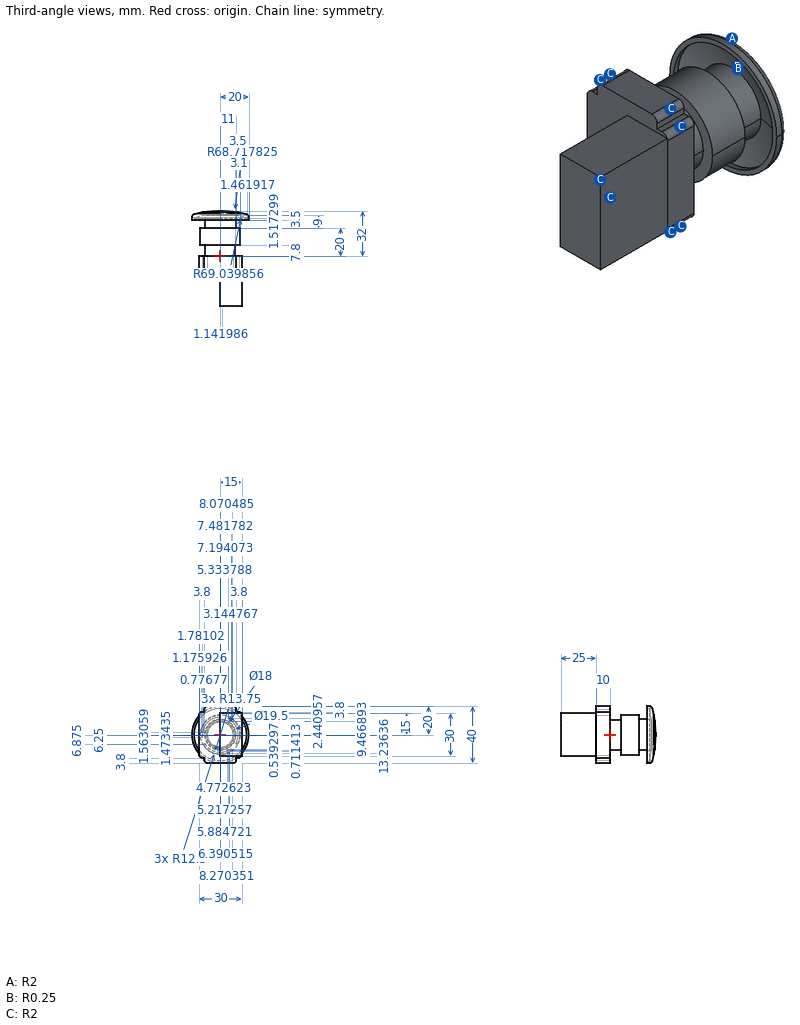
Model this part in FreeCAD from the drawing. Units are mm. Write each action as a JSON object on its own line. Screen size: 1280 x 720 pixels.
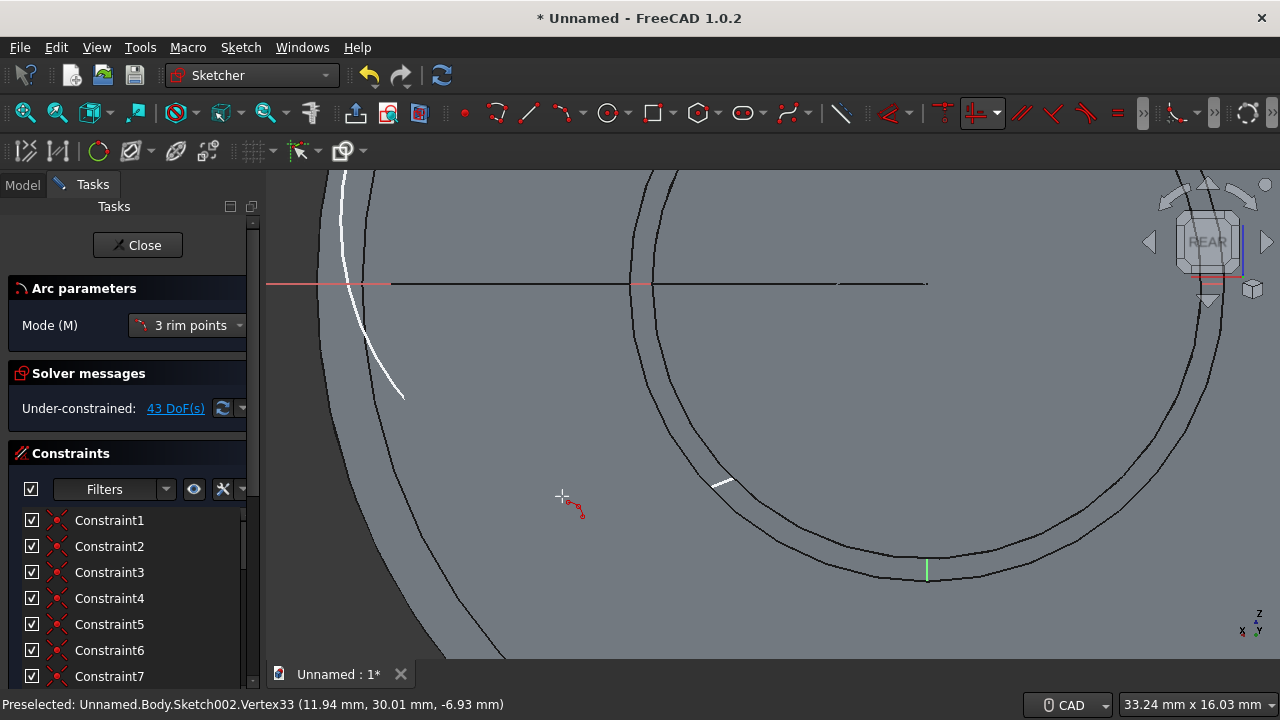
{"action": "scroll", "coordinate": [563, 495], "scroll_direction": "down", "scroll_amount": 5}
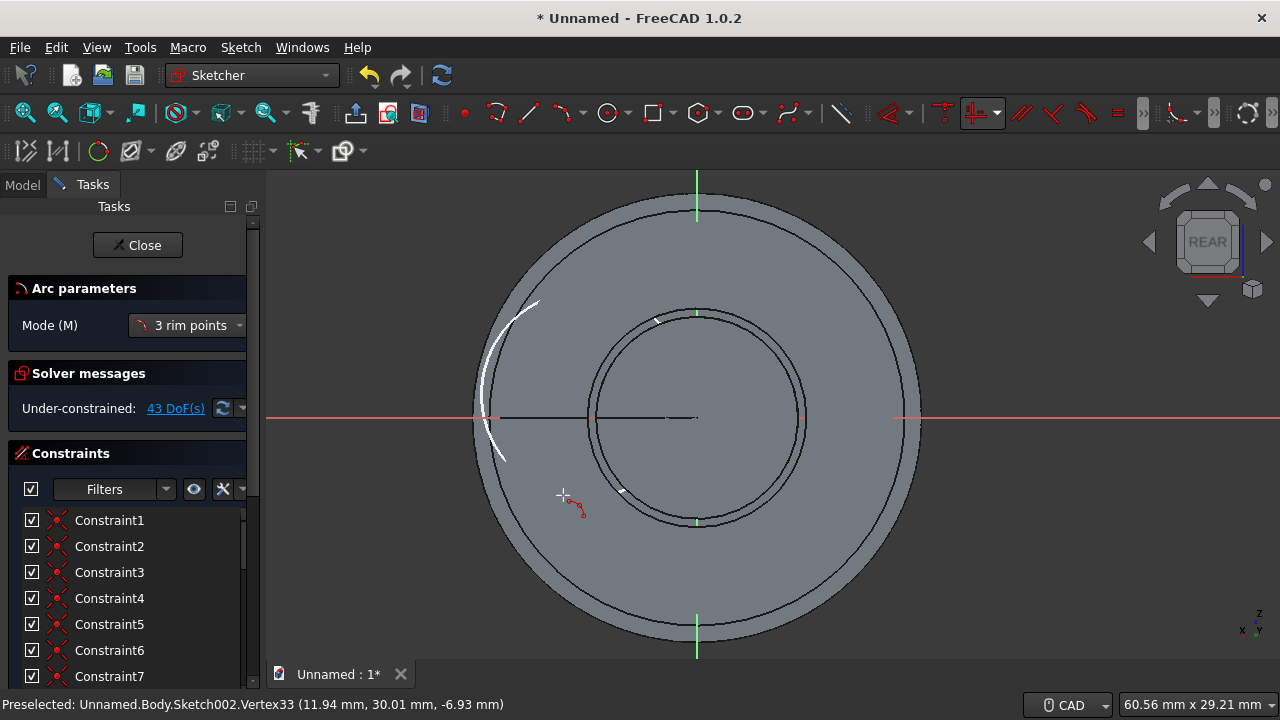
{"action": "left_click", "coordinate": [546, 386]}
{"action": "key", "text": "Escape"}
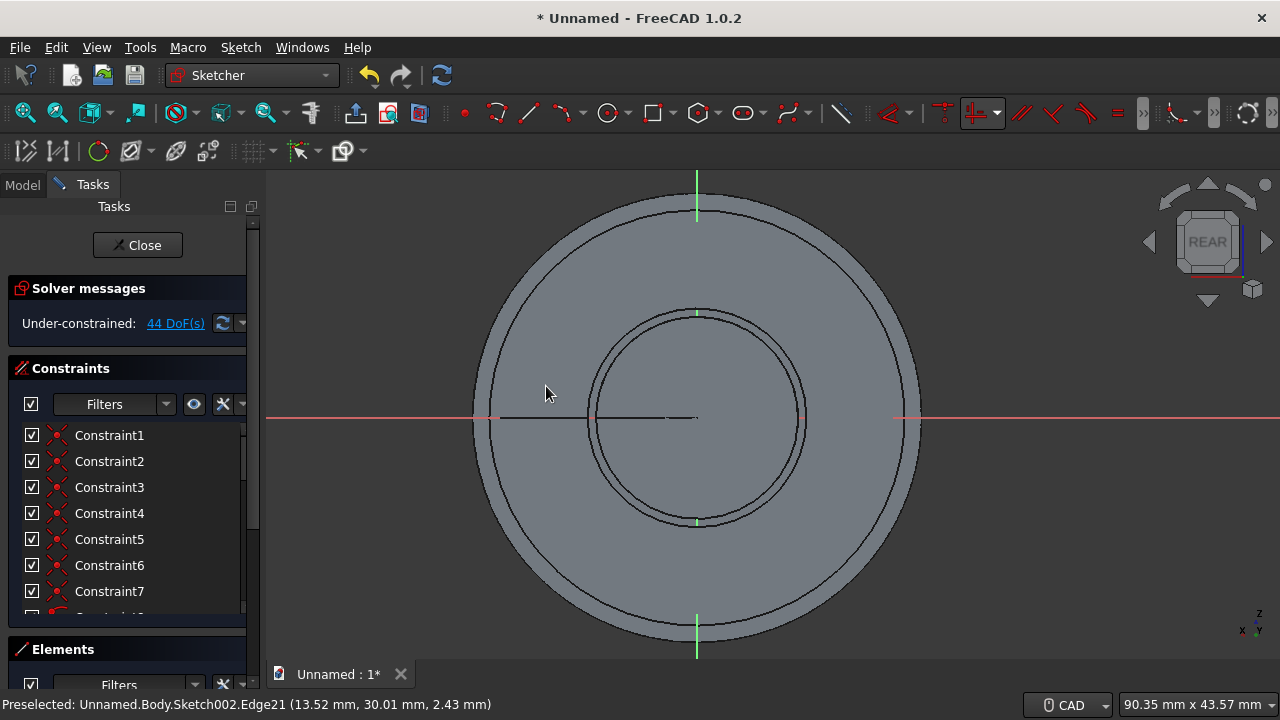
{"action": "scroll", "coordinate": [701, 270], "scroll_direction": "up", "scroll_amount": 5}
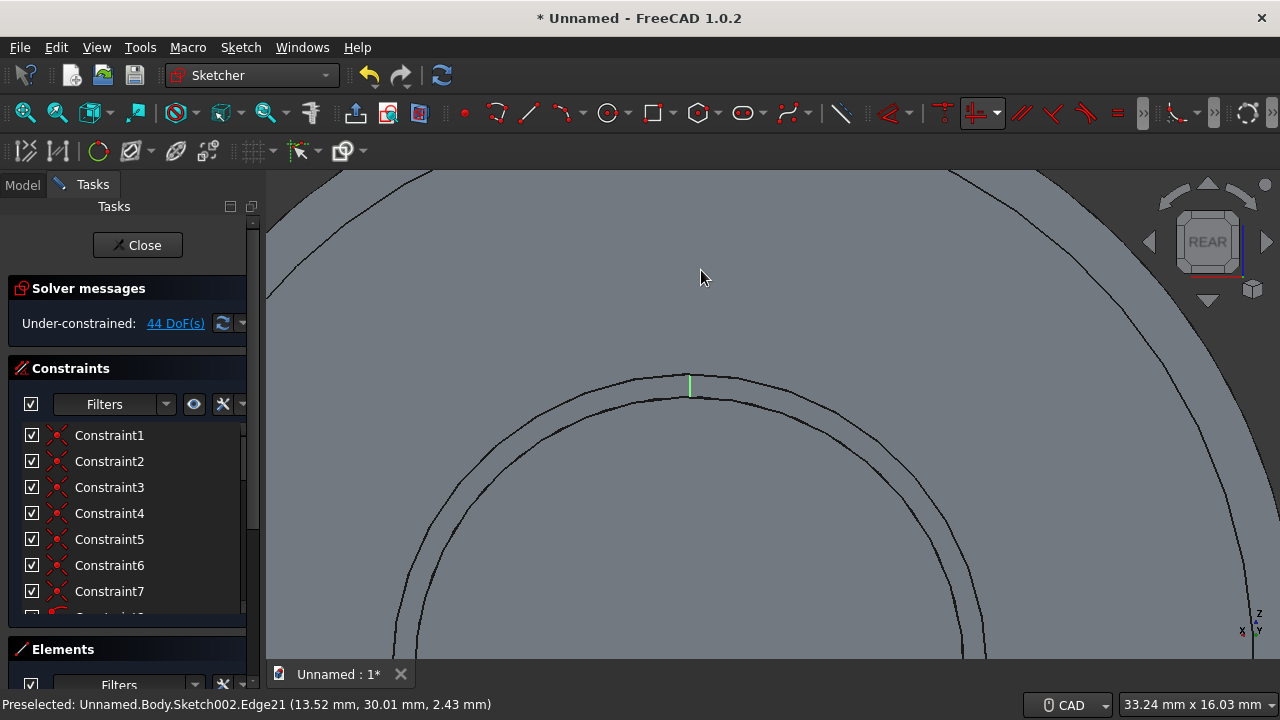
{"action": "left_click", "coordinate": [699, 269]}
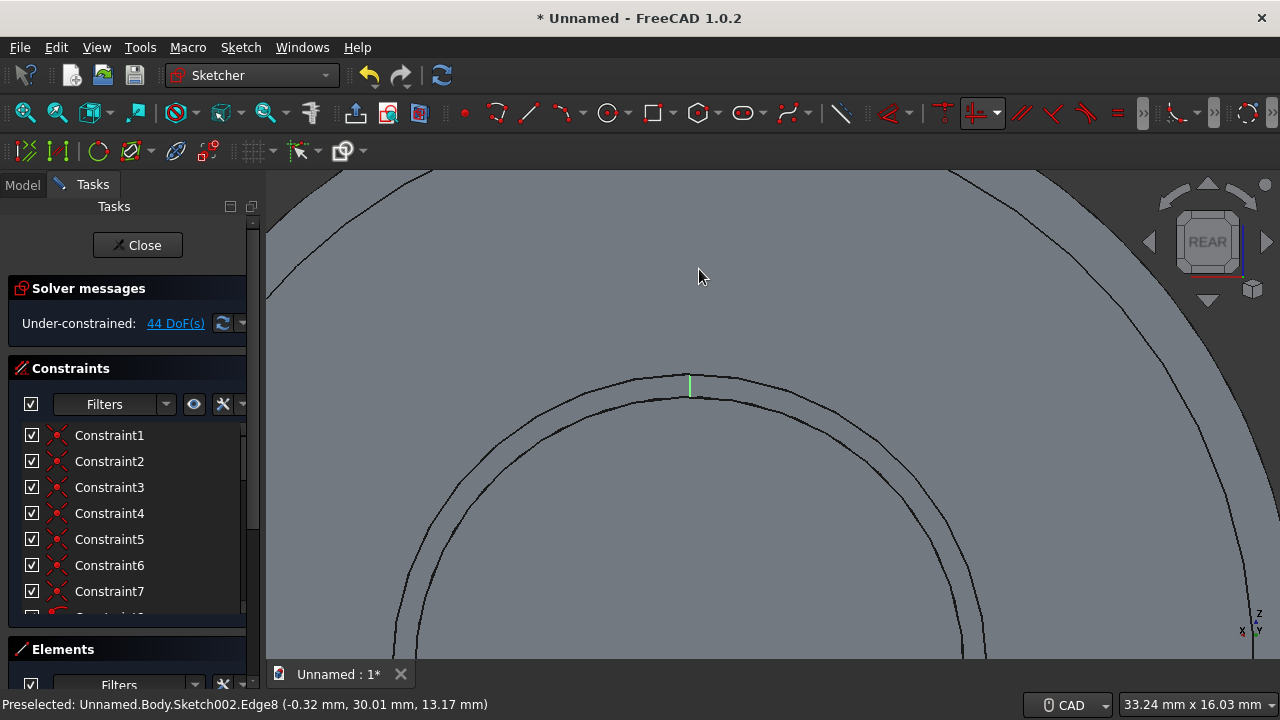
{"action": "left_click", "coordinate": [1000, 114]}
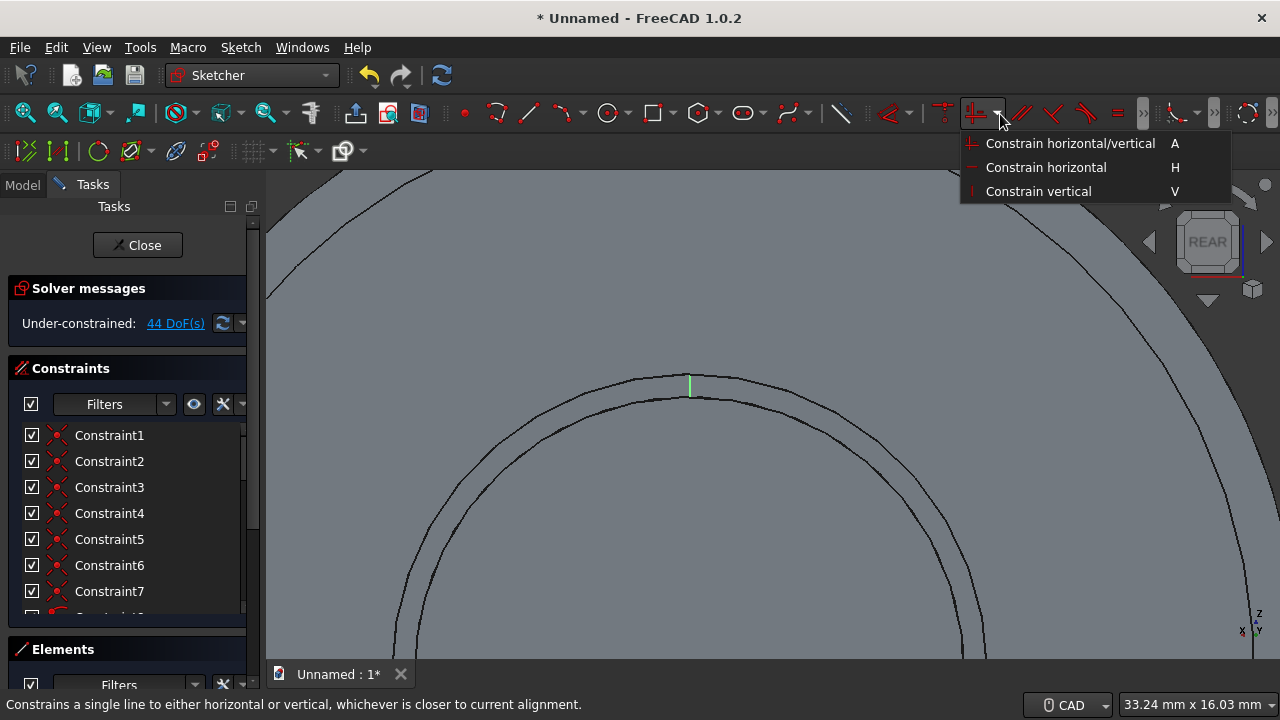
{"action": "left_click", "coordinate": [1096, 191]}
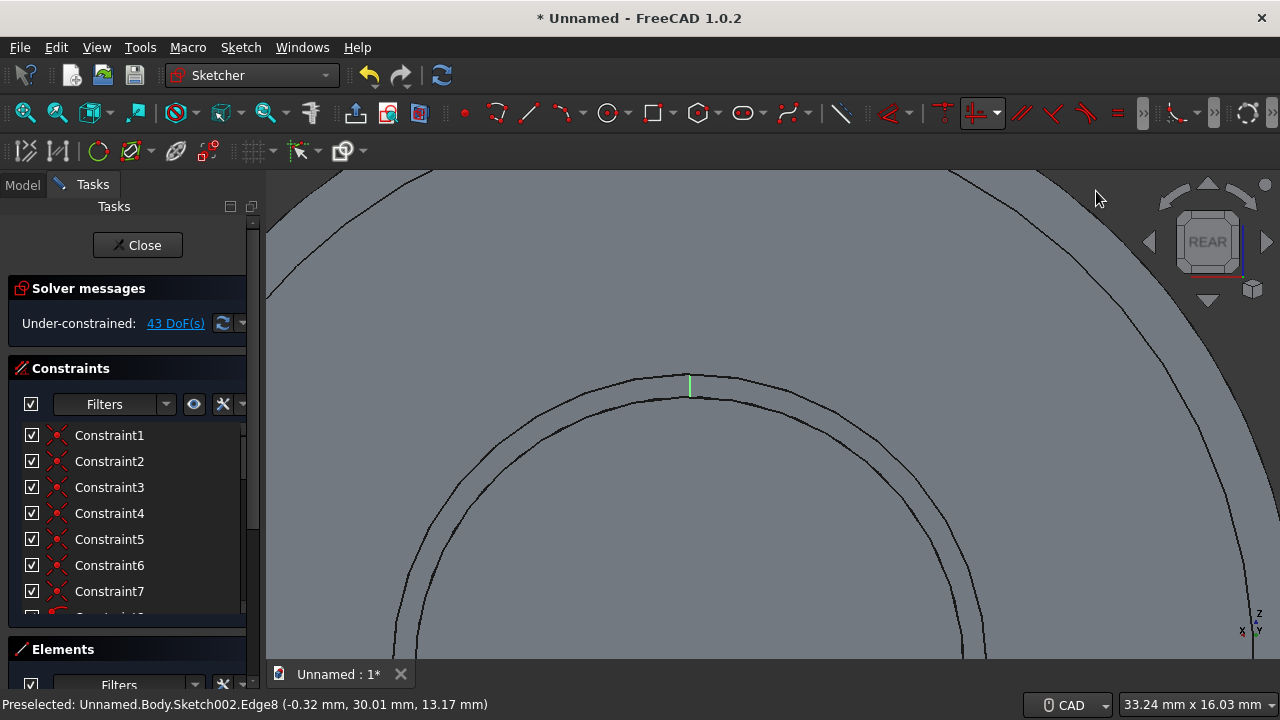
{"action": "scroll", "coordinate": [701, 269], "scroll_direction": "down", "scroll_amount": 5}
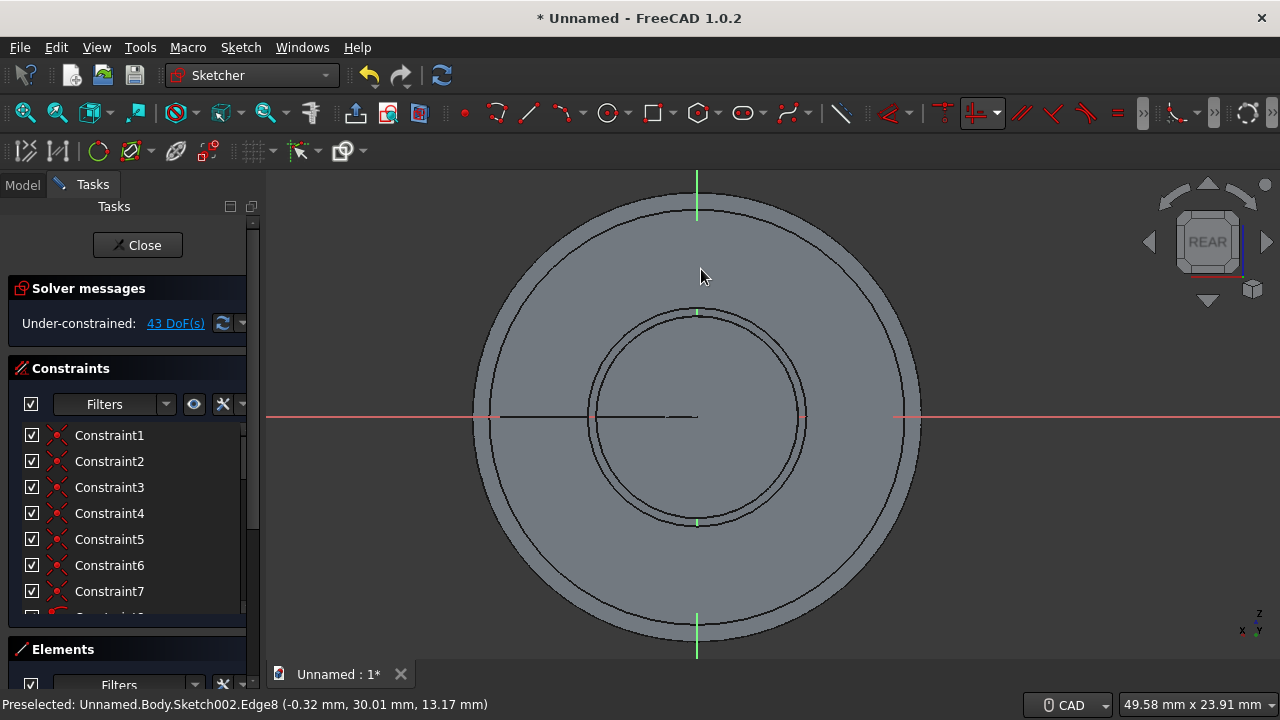
{"action": "left_click", "coordinate": [776, 534]}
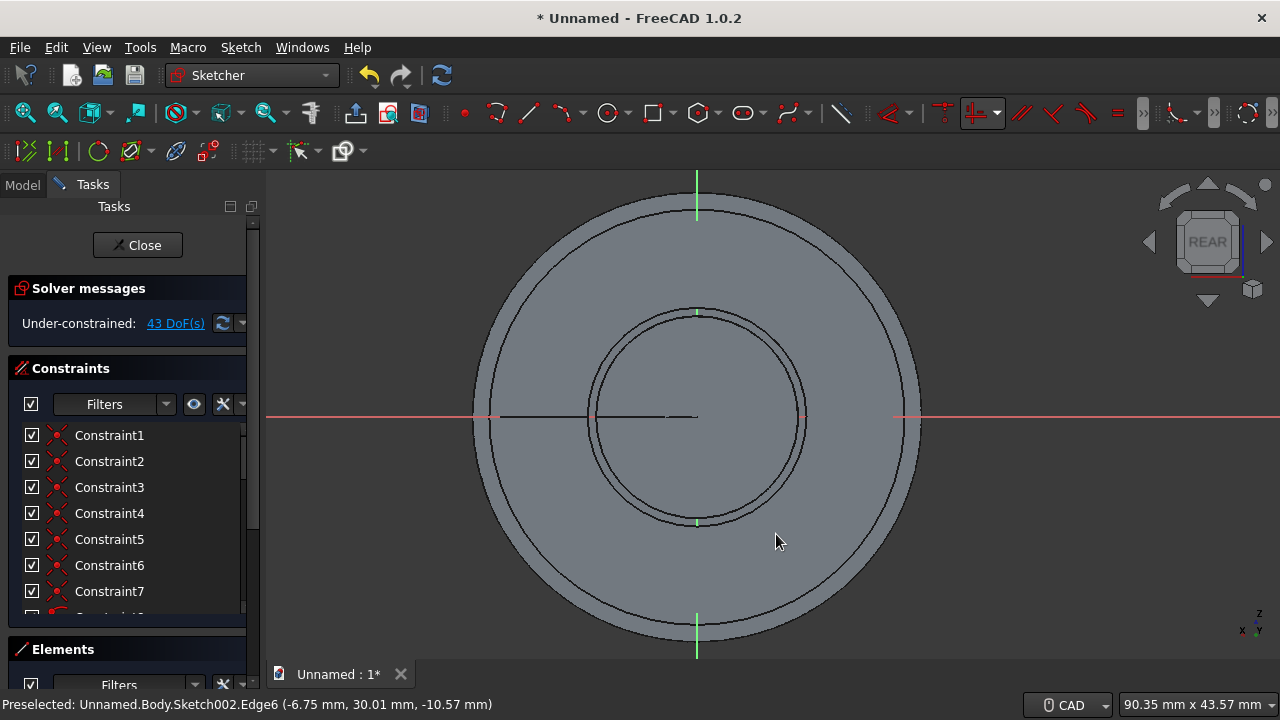
{"action": "left_click", "coordinate": [697, 572]}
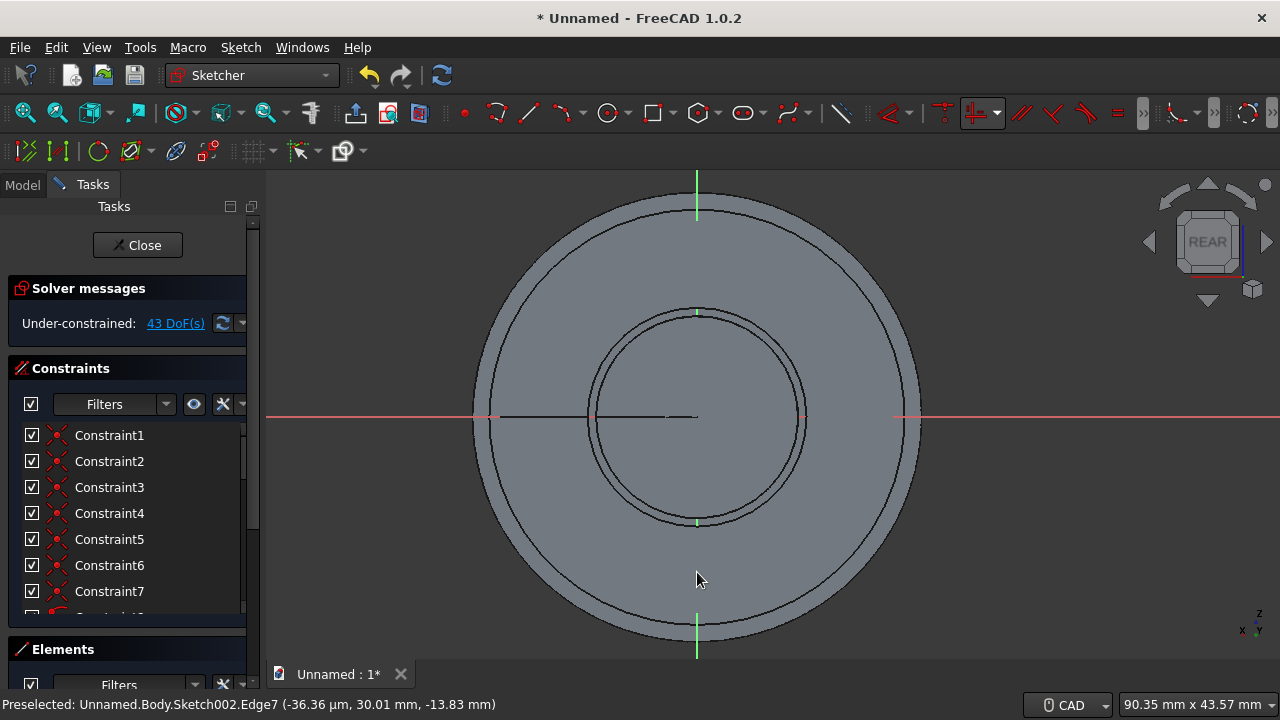
{"action": "left_click", "coordinate": [944, 114]}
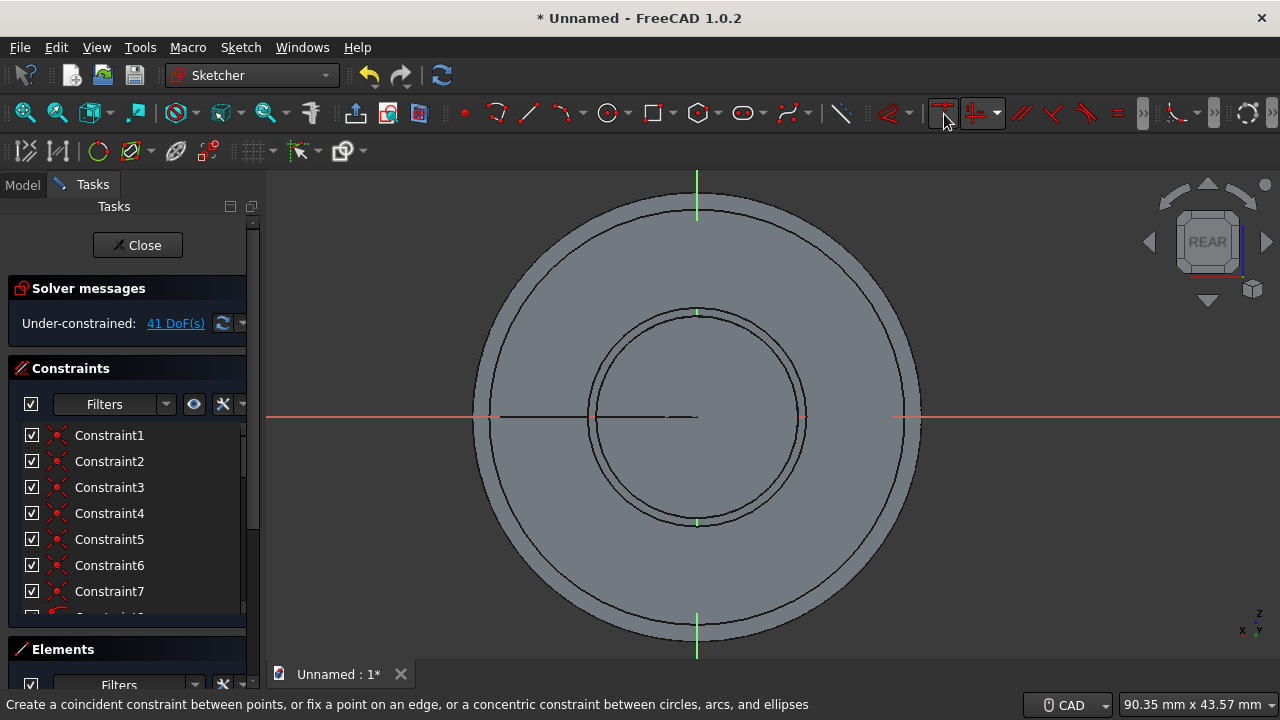
{"action": "left_click", "coordinate": [699, 559]}